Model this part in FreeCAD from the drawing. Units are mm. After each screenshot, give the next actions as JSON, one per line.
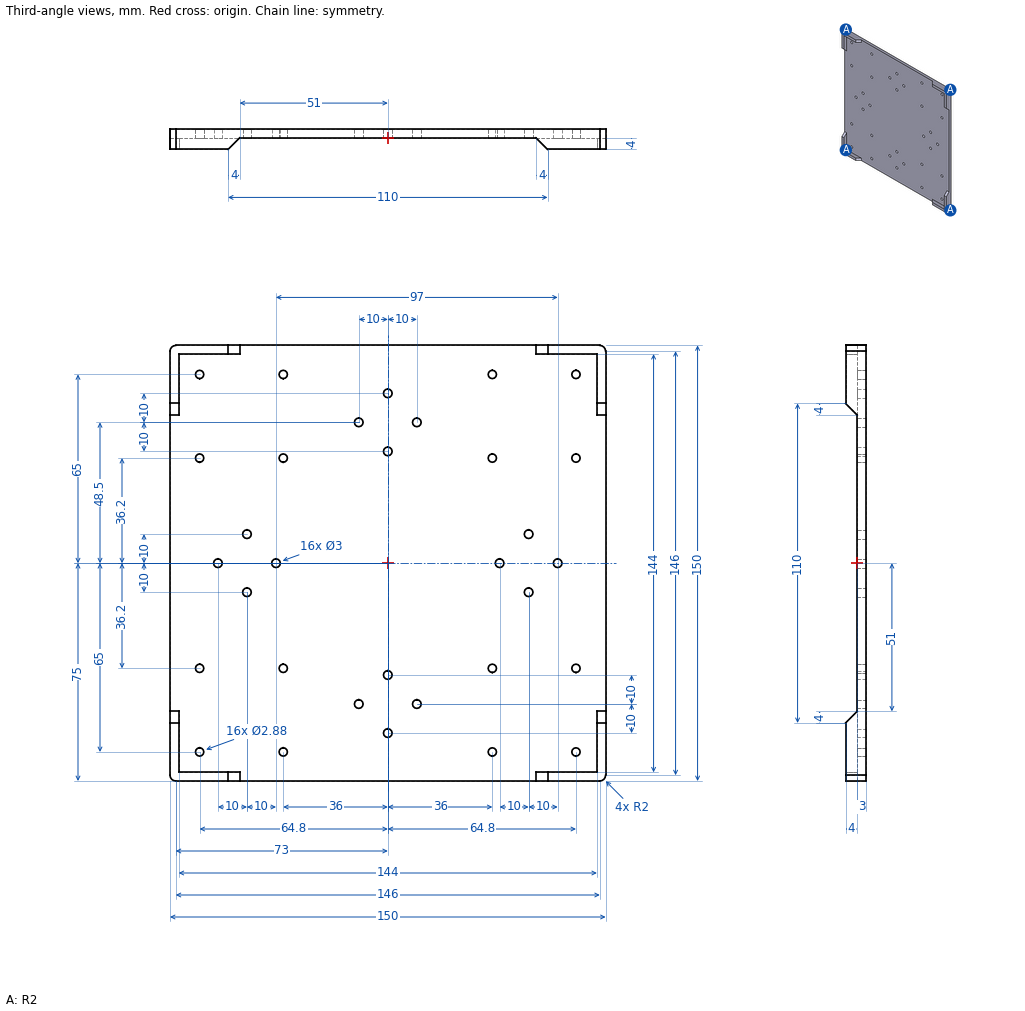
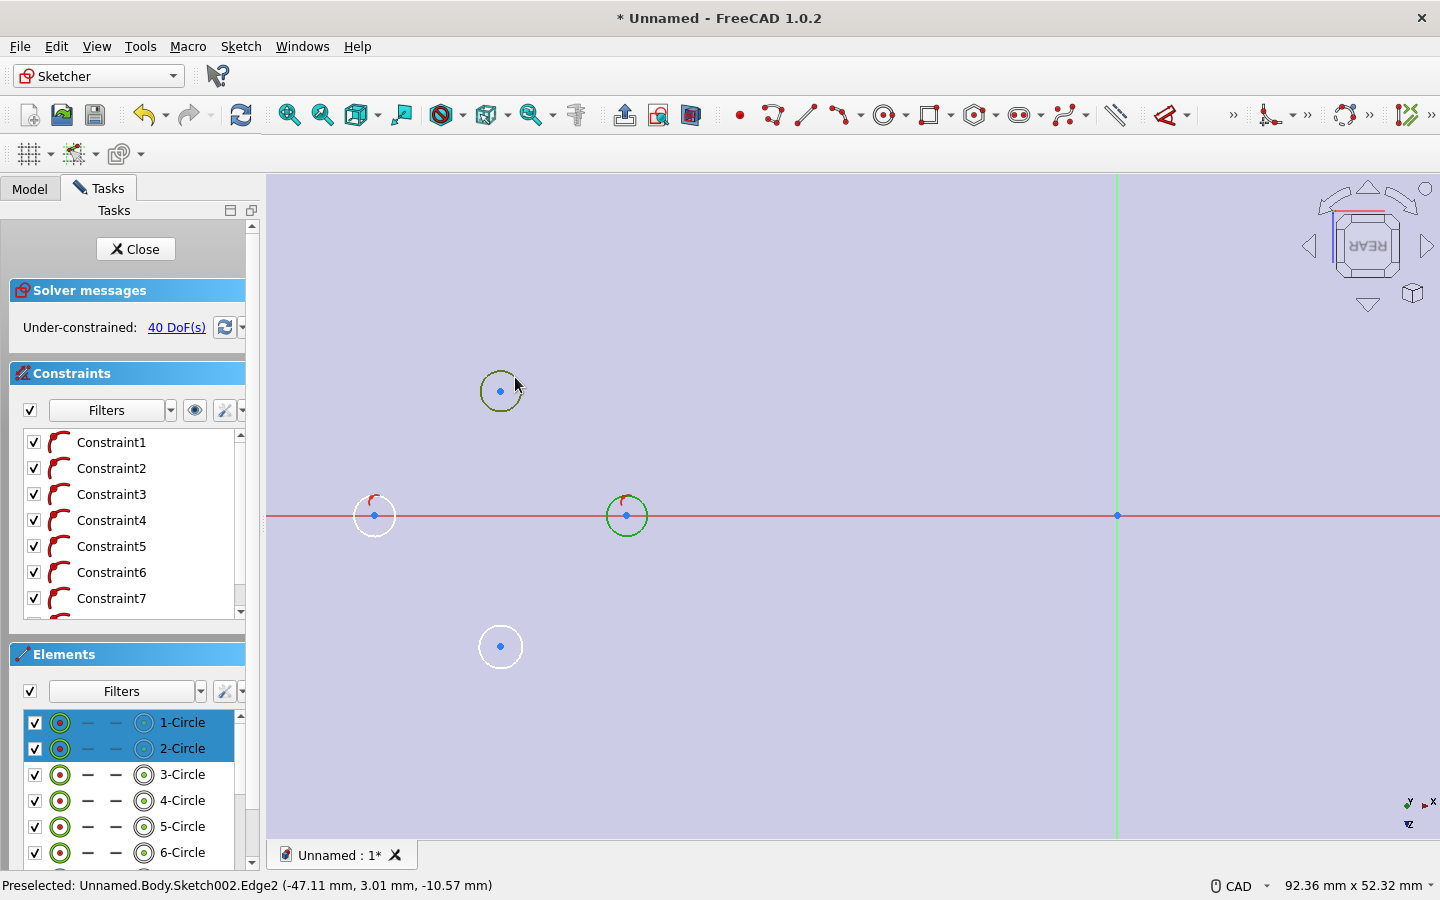
{"action": "left_click", "coordinate": [389, 501]}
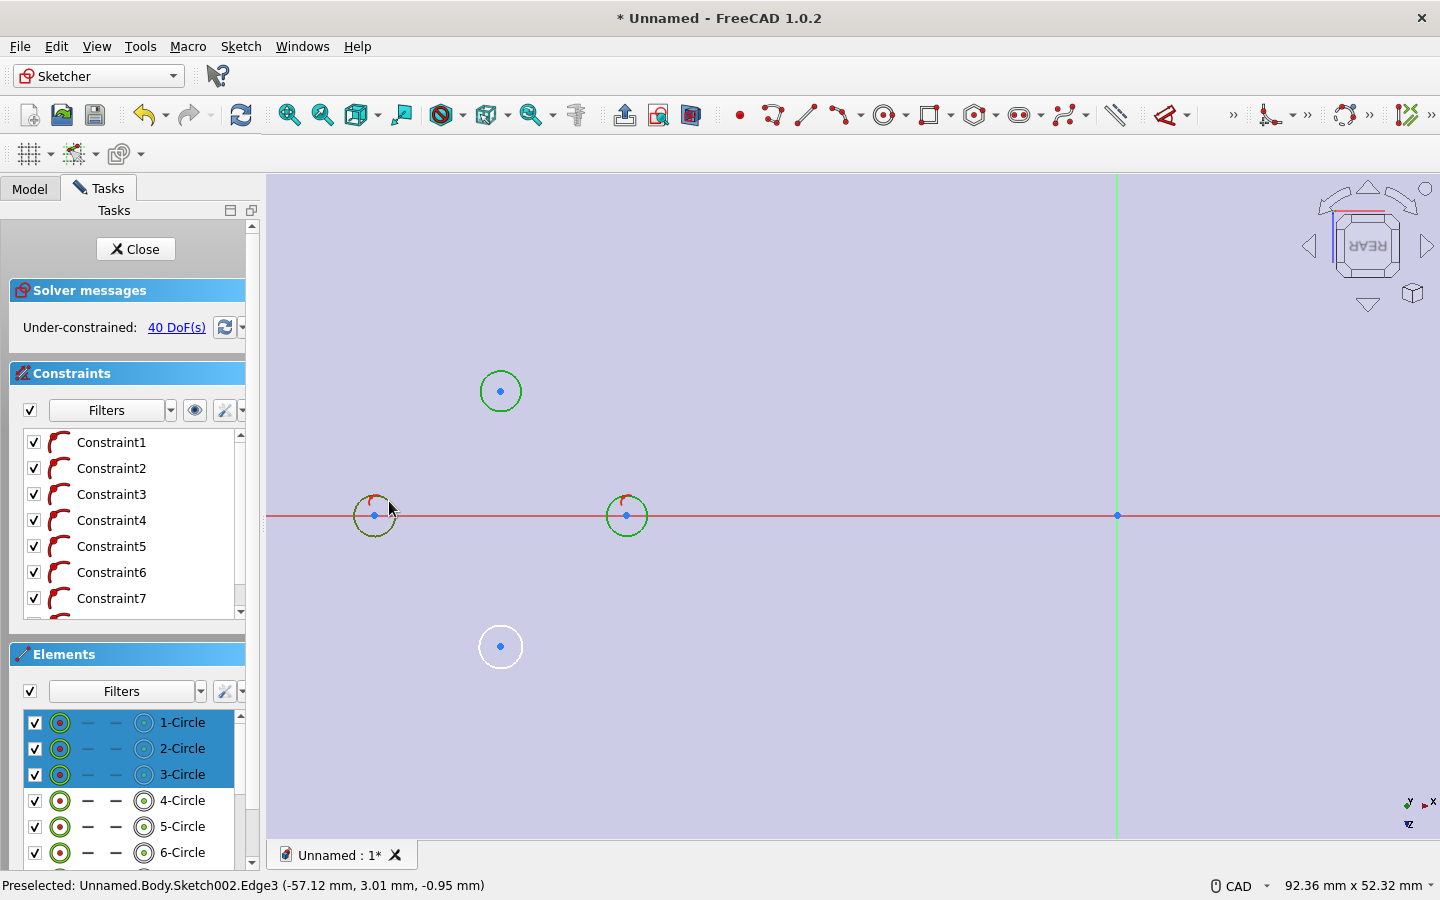
{"action": "left_click", "coordinate": [516, 632]}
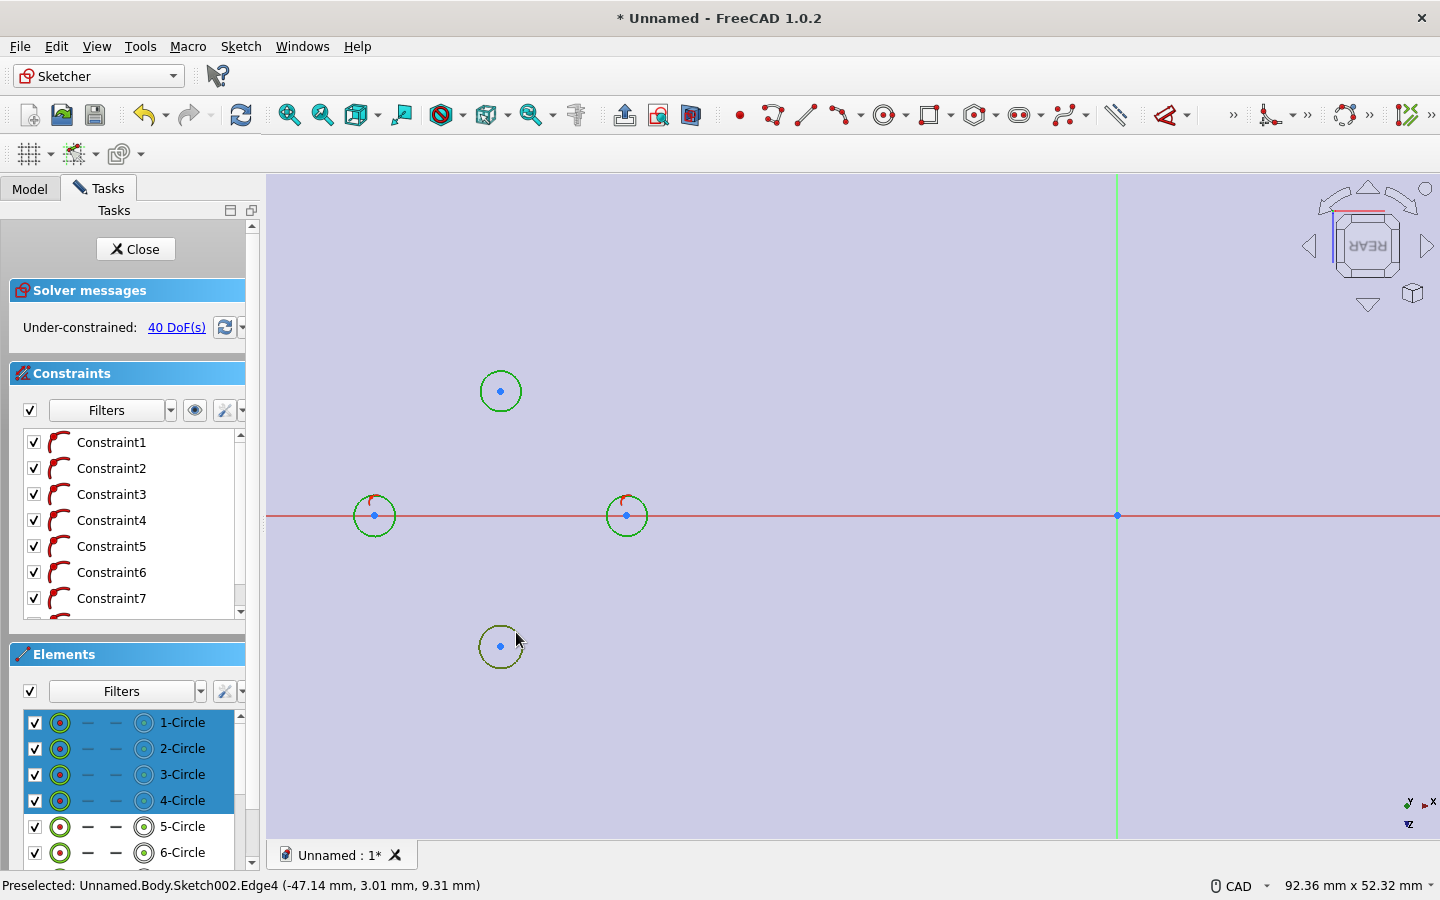
{"action": "scroll", "coordinate": [641, 502], "scroll_direction": "down", "scroll_amount": 6}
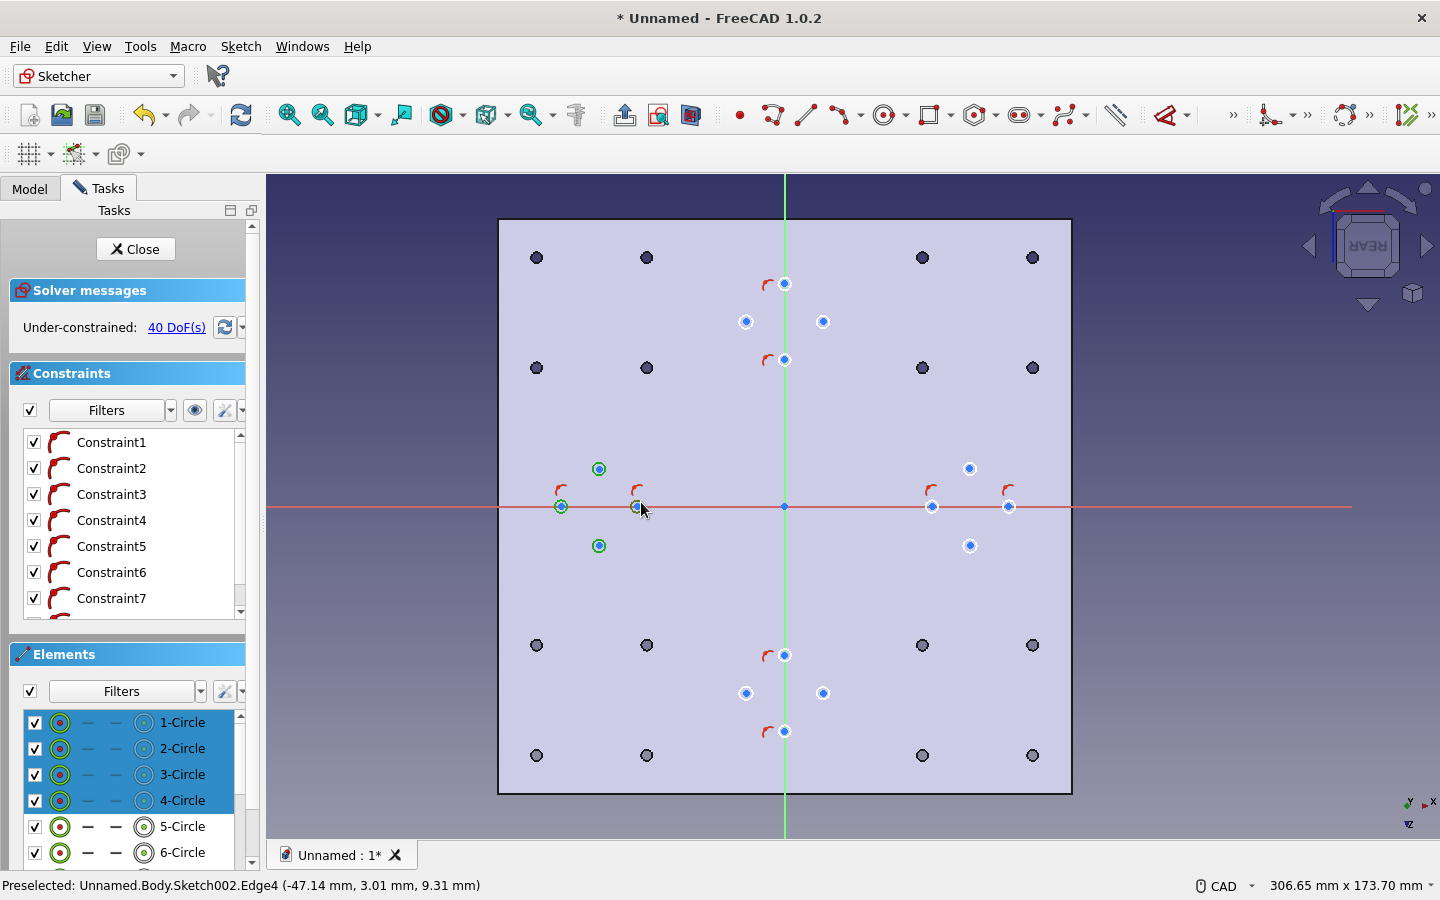
{"action": "scroll", "coordinate": [751, 689], "scroll_direction": "up", "scroll_amount": 4}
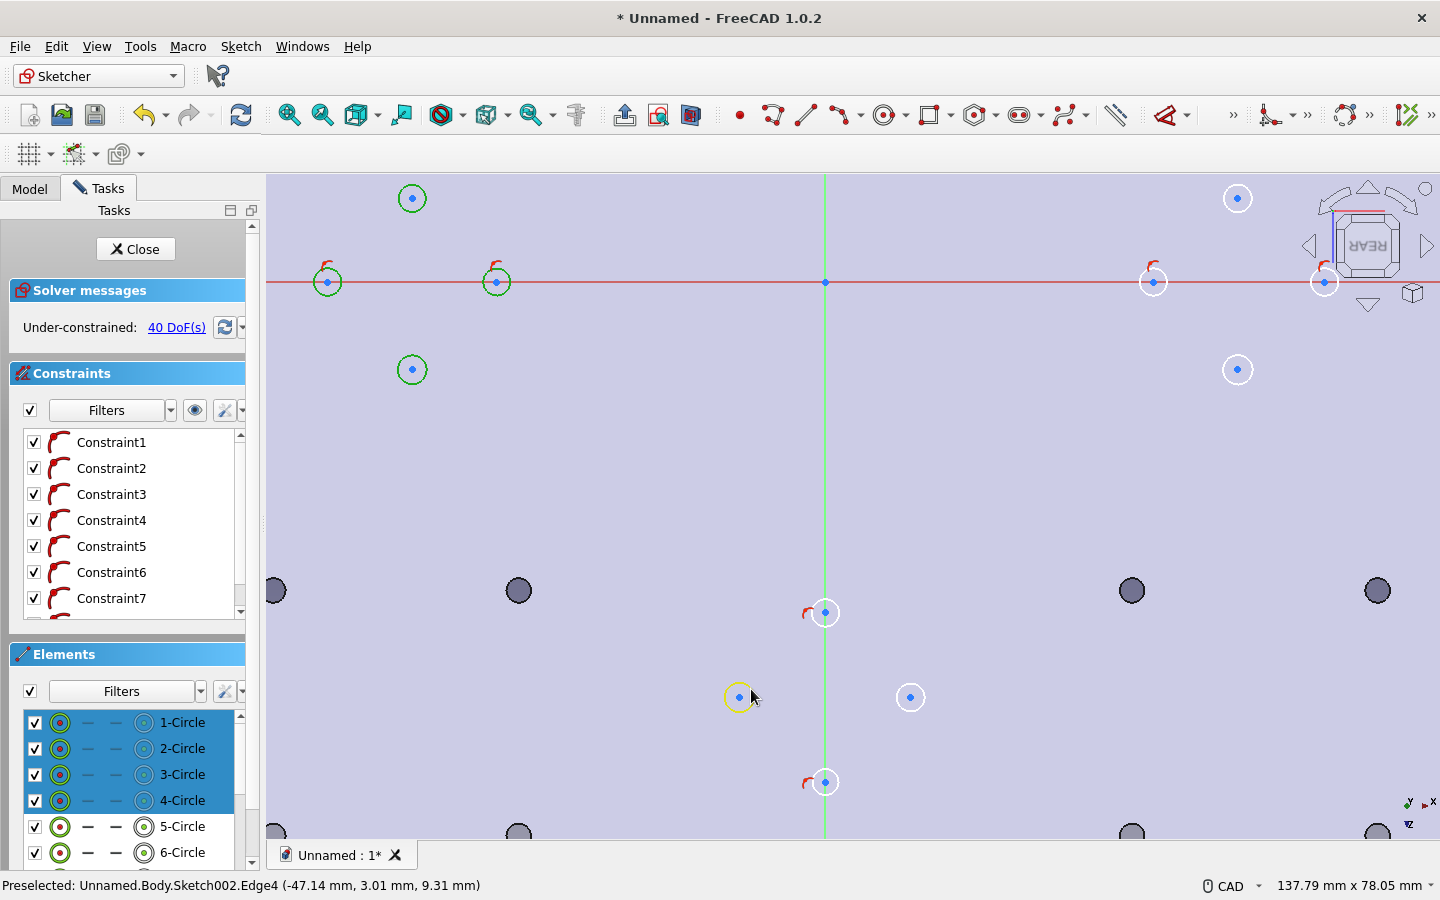
{"action": "left_click", "coordinate": [750, 687]}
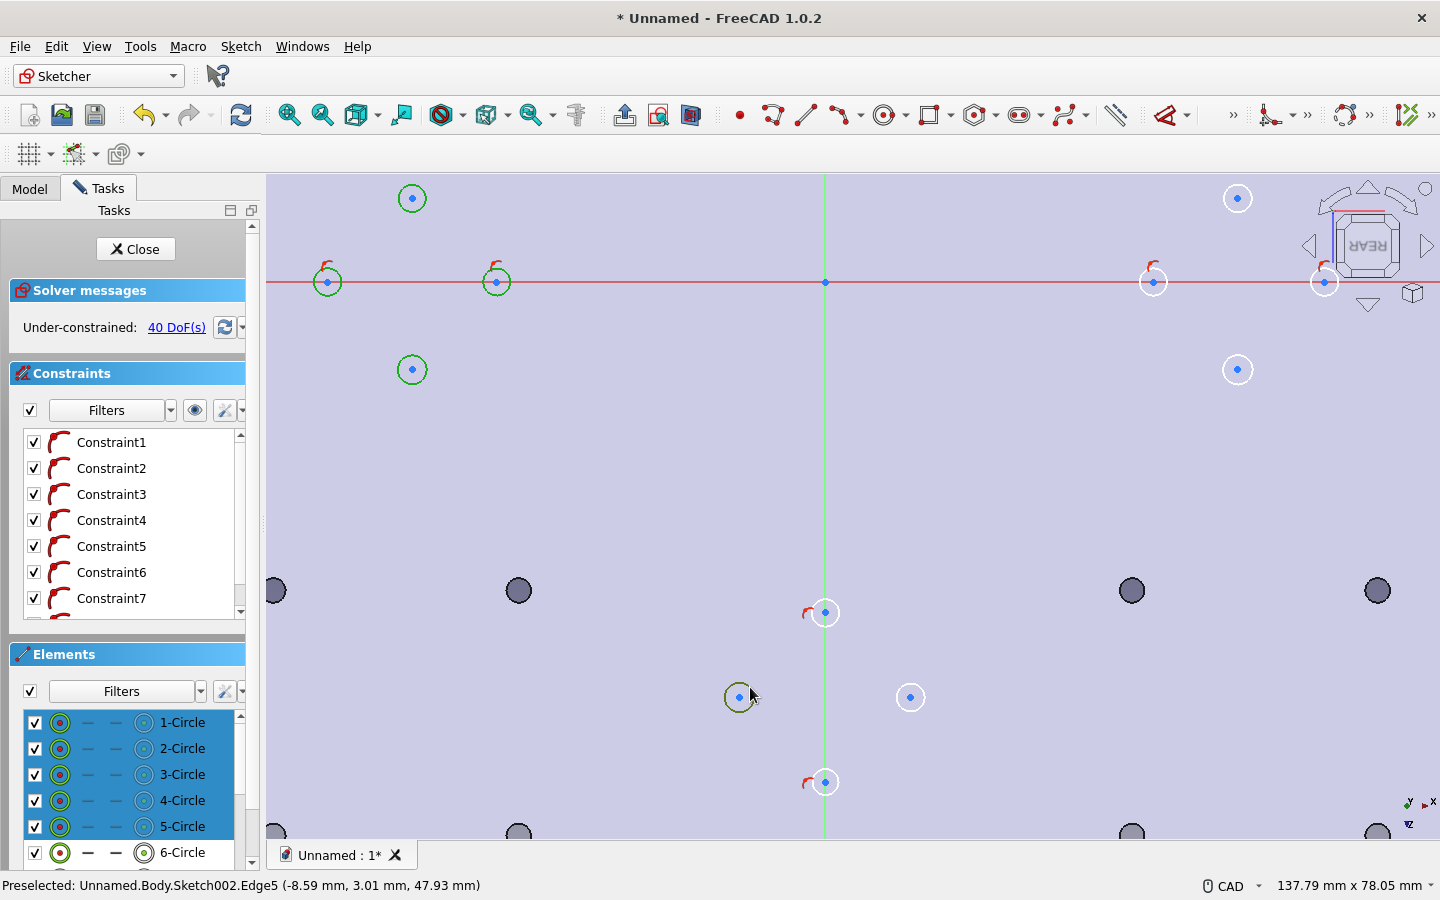
{"action": "scroll", "coordinate": [835, 773], "scroll_direction": "up", "scroll_amount": 3}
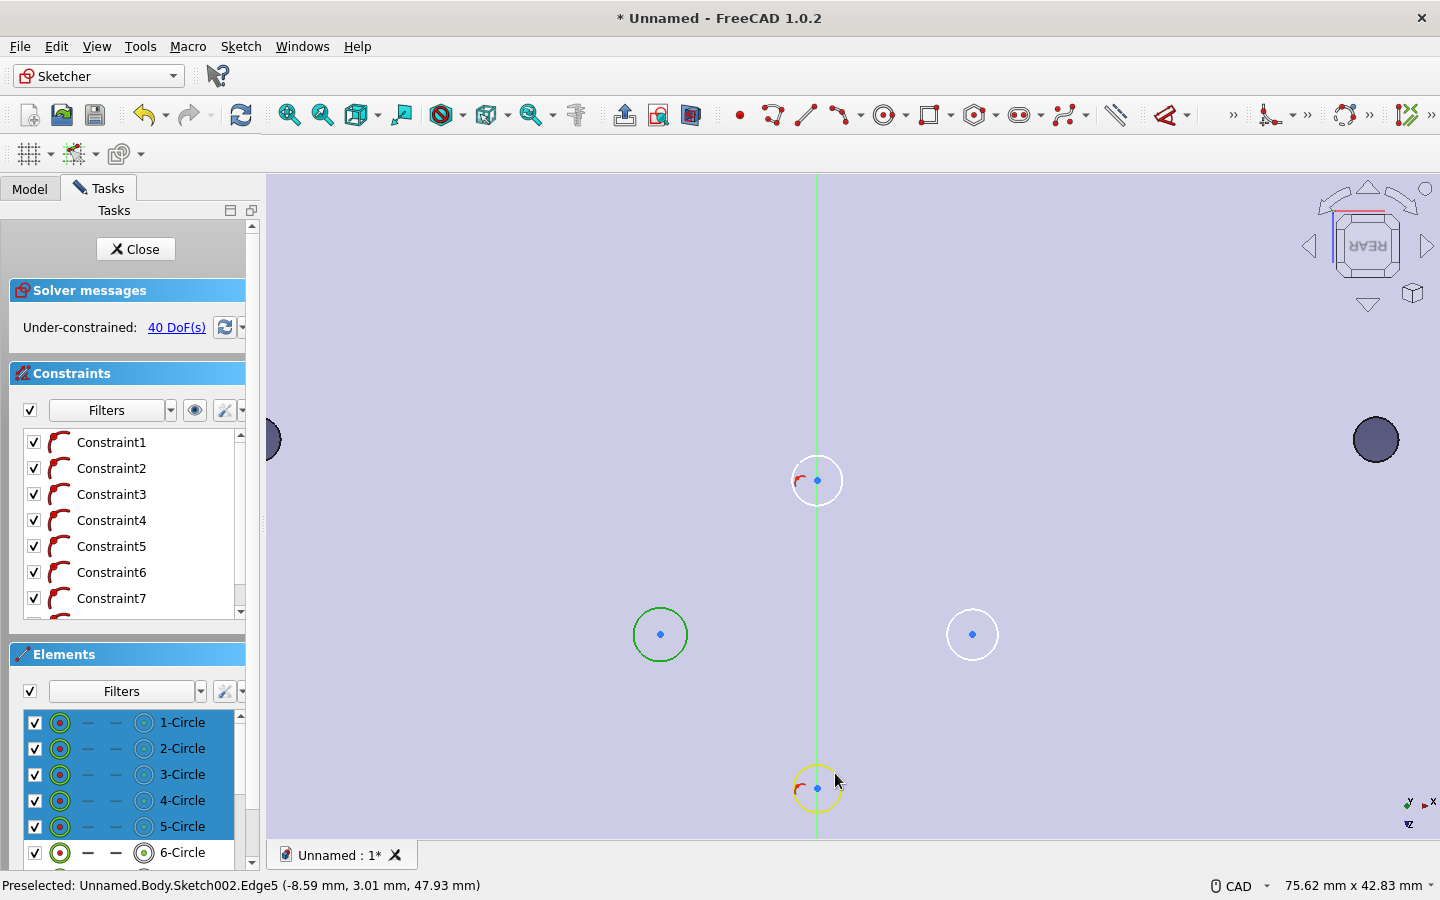
{"action": "left_click", "coordinate": [834, 772]}